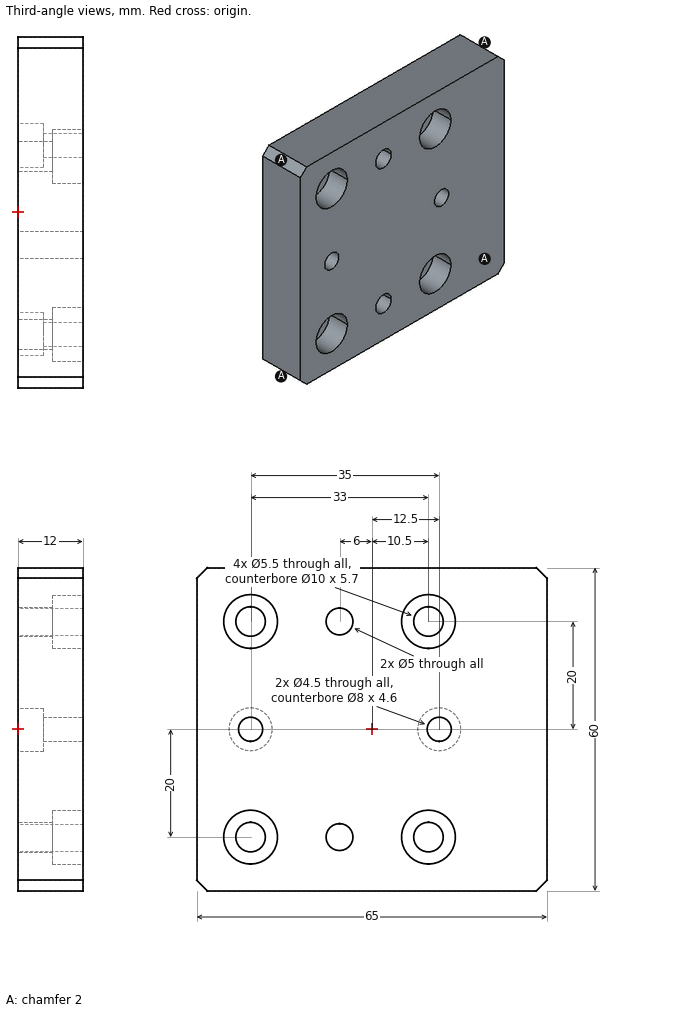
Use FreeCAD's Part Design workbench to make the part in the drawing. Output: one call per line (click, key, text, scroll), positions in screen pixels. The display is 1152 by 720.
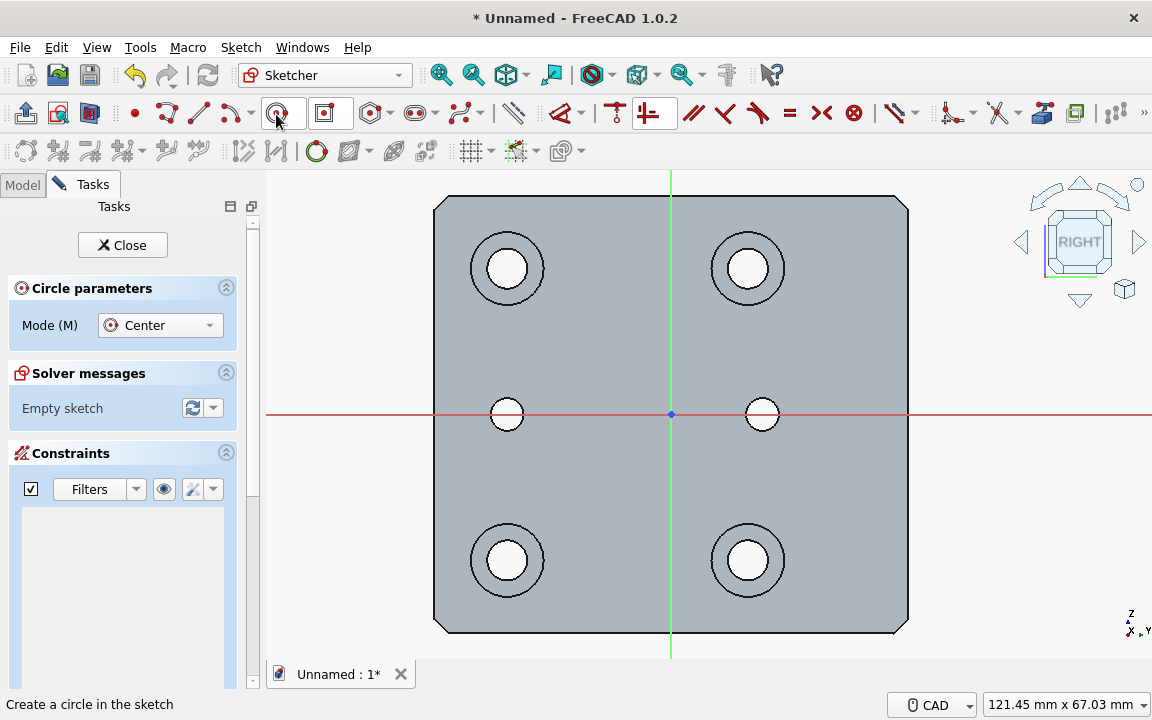
scroll(628, 269, up, 2)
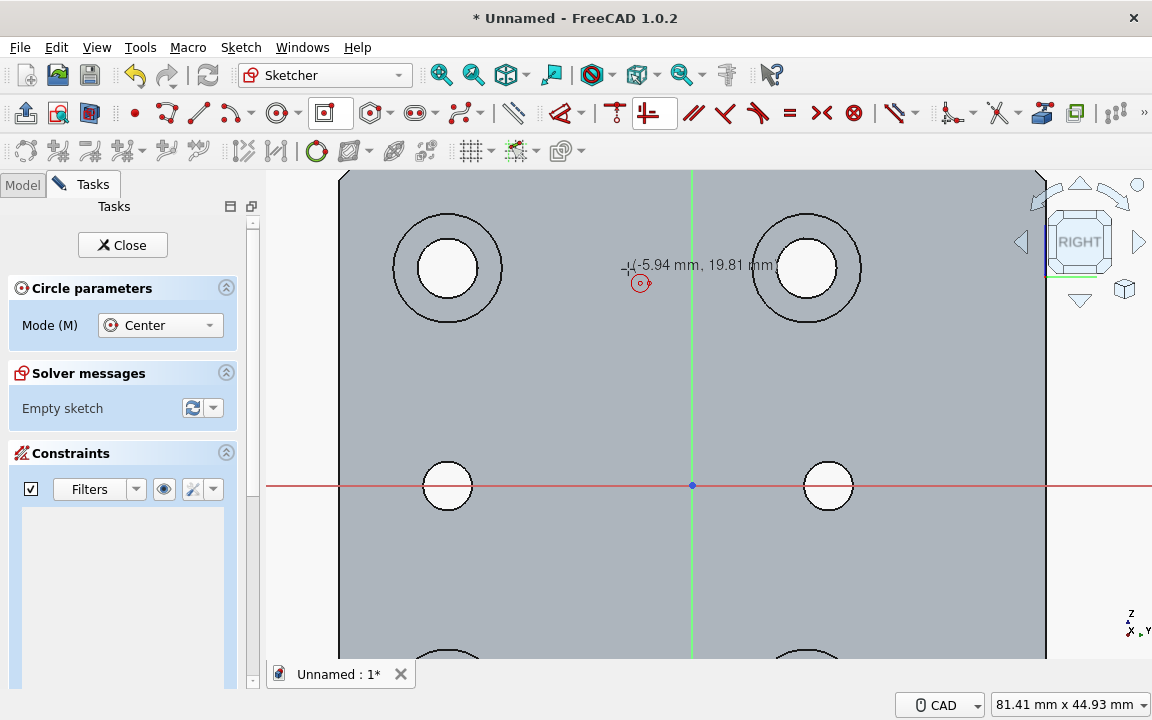
click(627, 268)
click(646, 249)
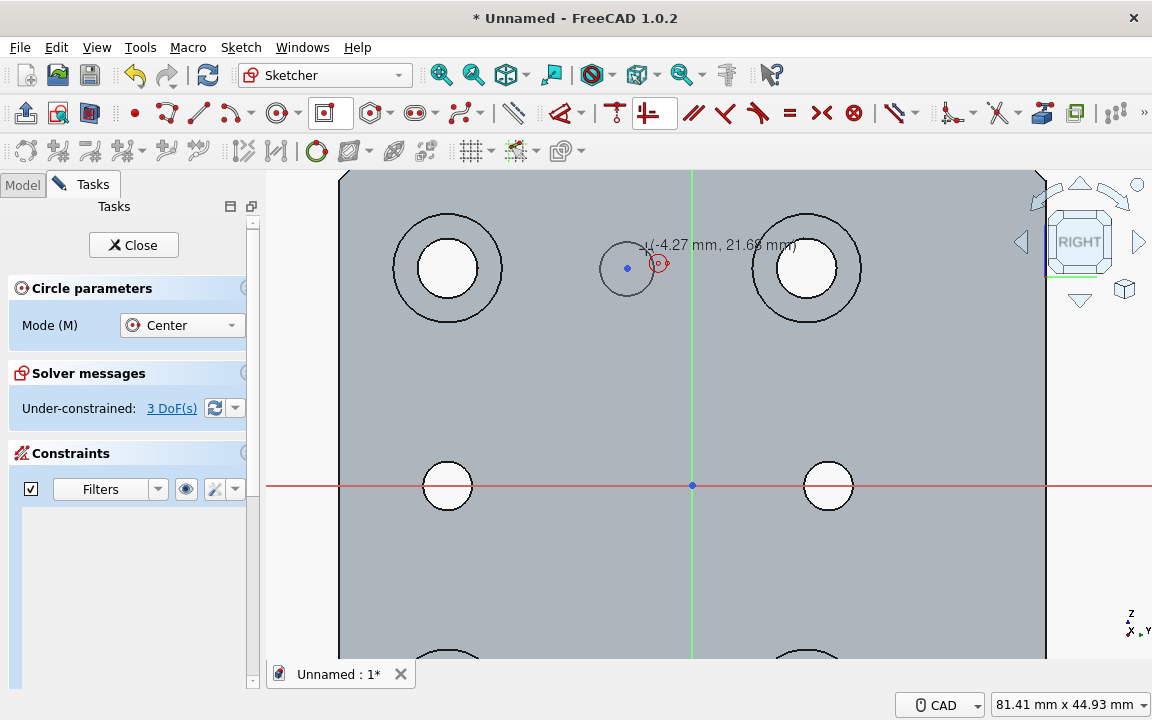
scroll(629, 269, down, 2)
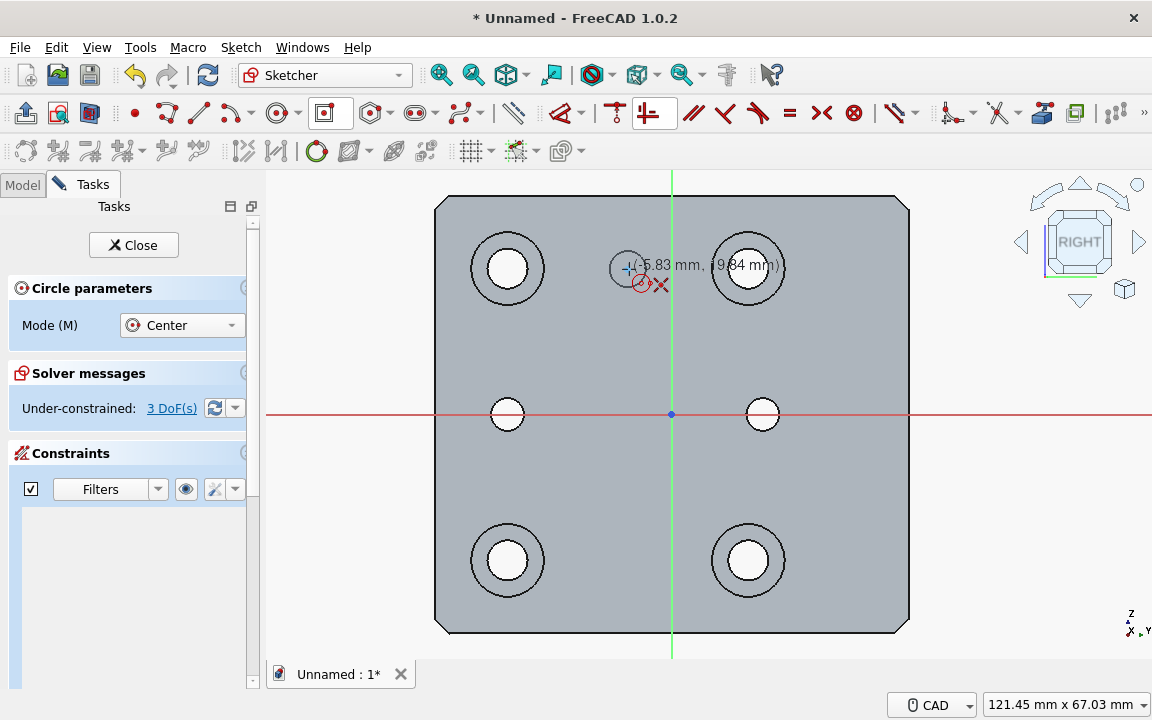
scroll(628, 560, up, 2)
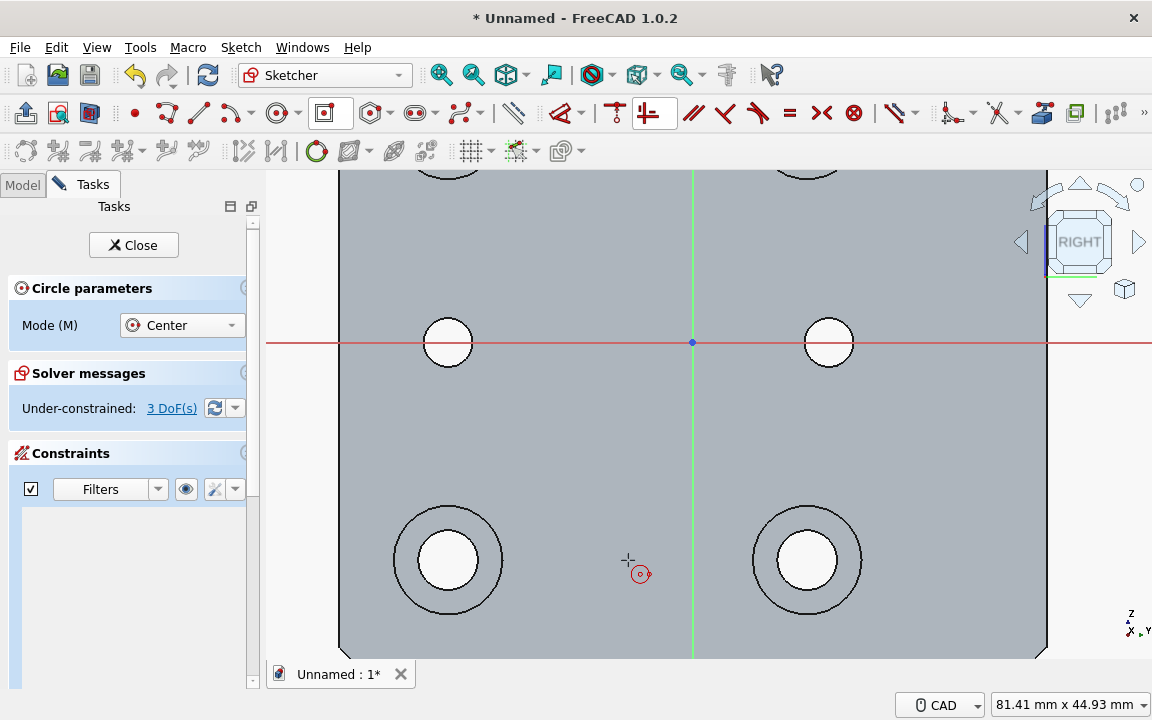
click(628, 560)
click(647, 541)
key(Escape)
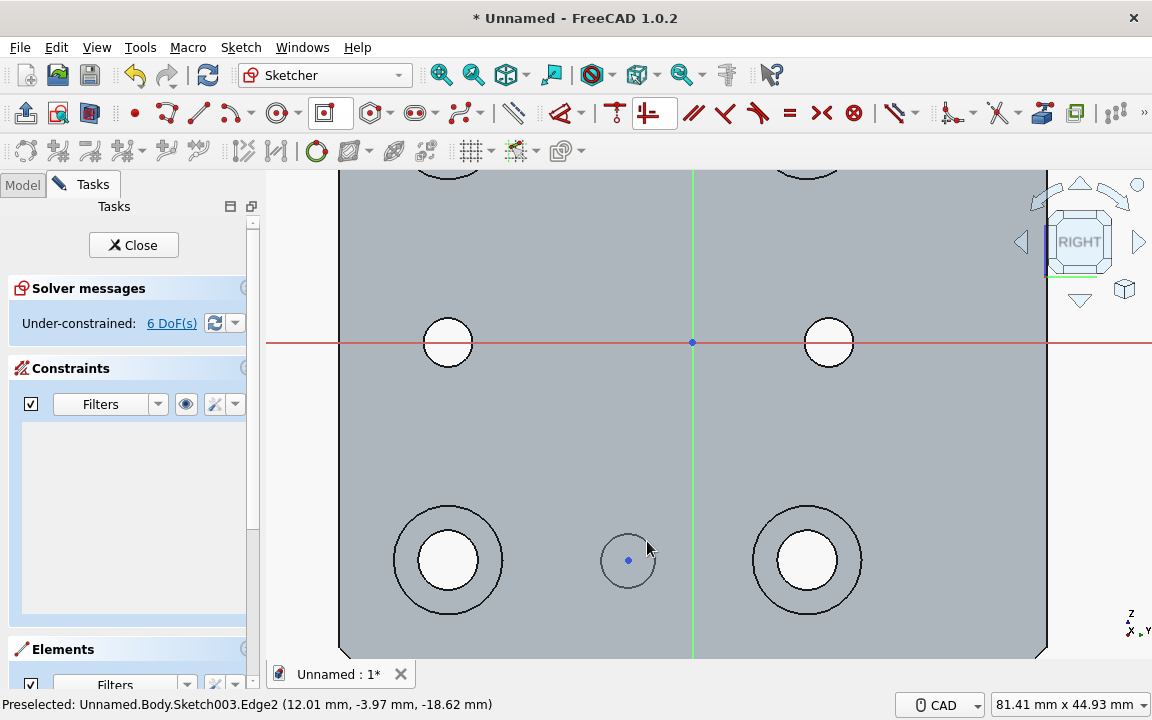
scroll(628, 561, down, 2)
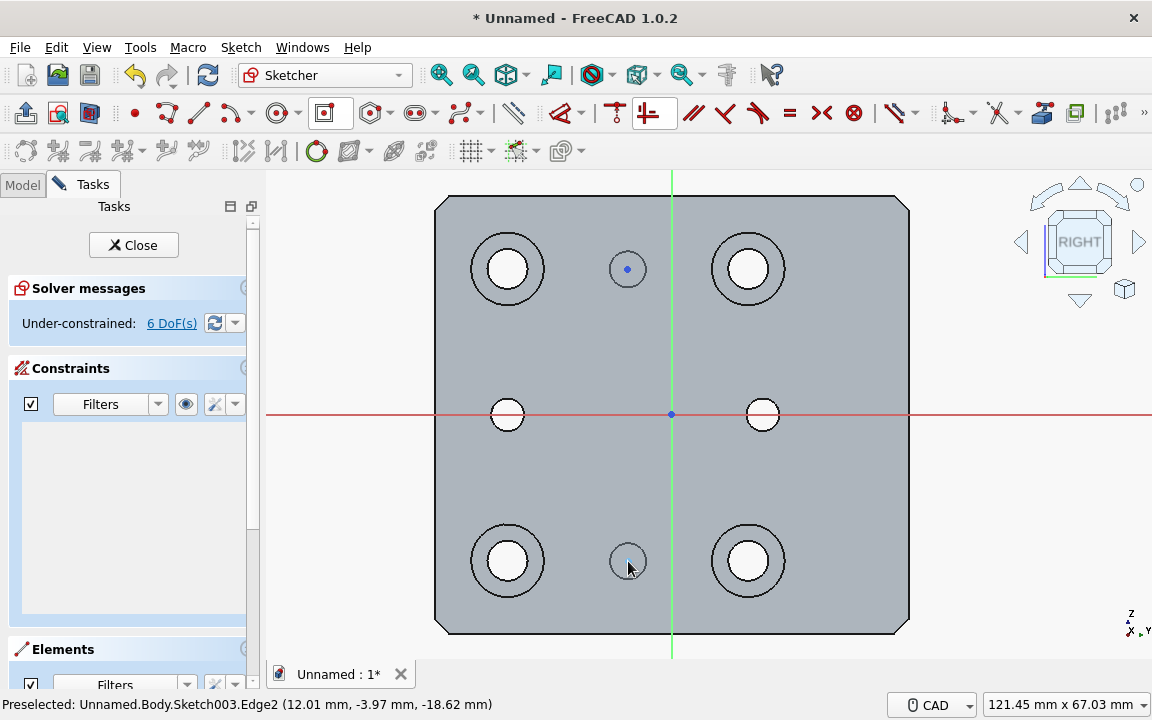
click(640, 257)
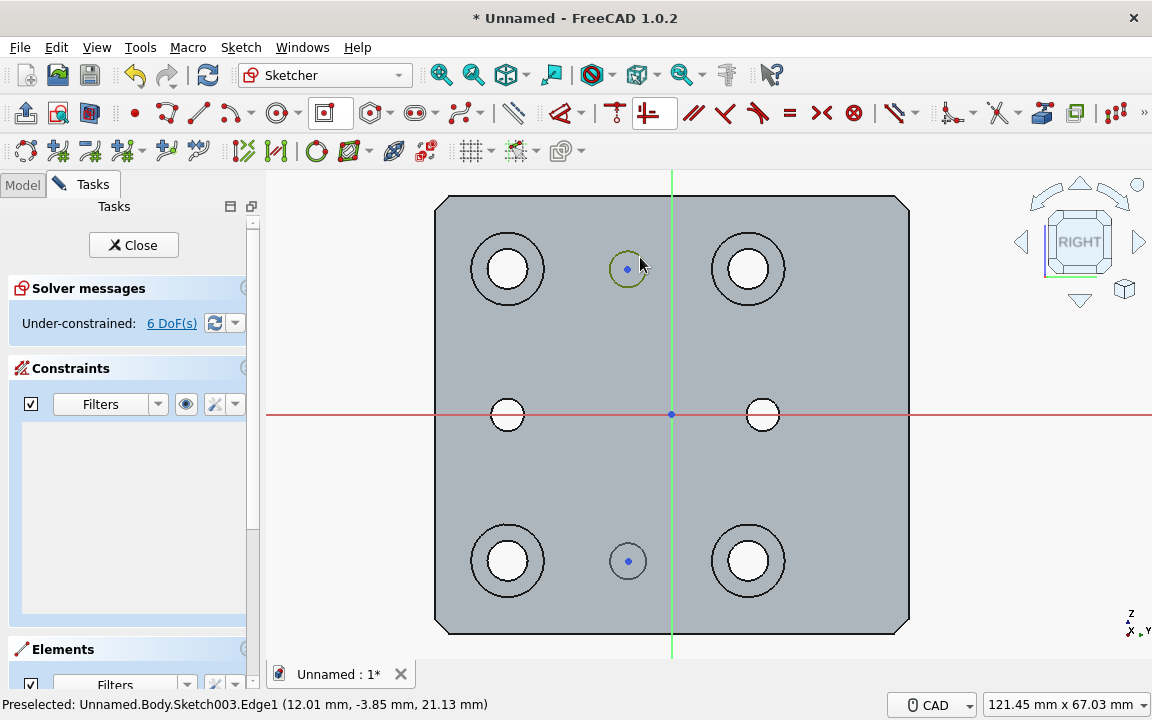
click(641, 548)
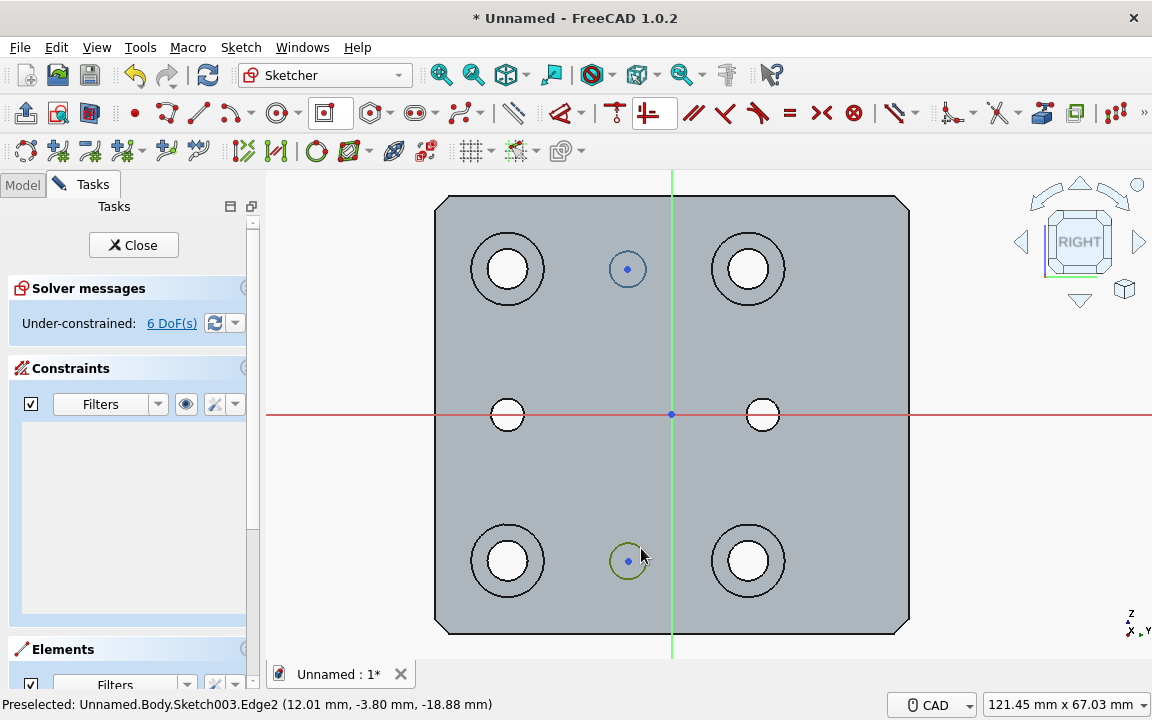
click(790, 114)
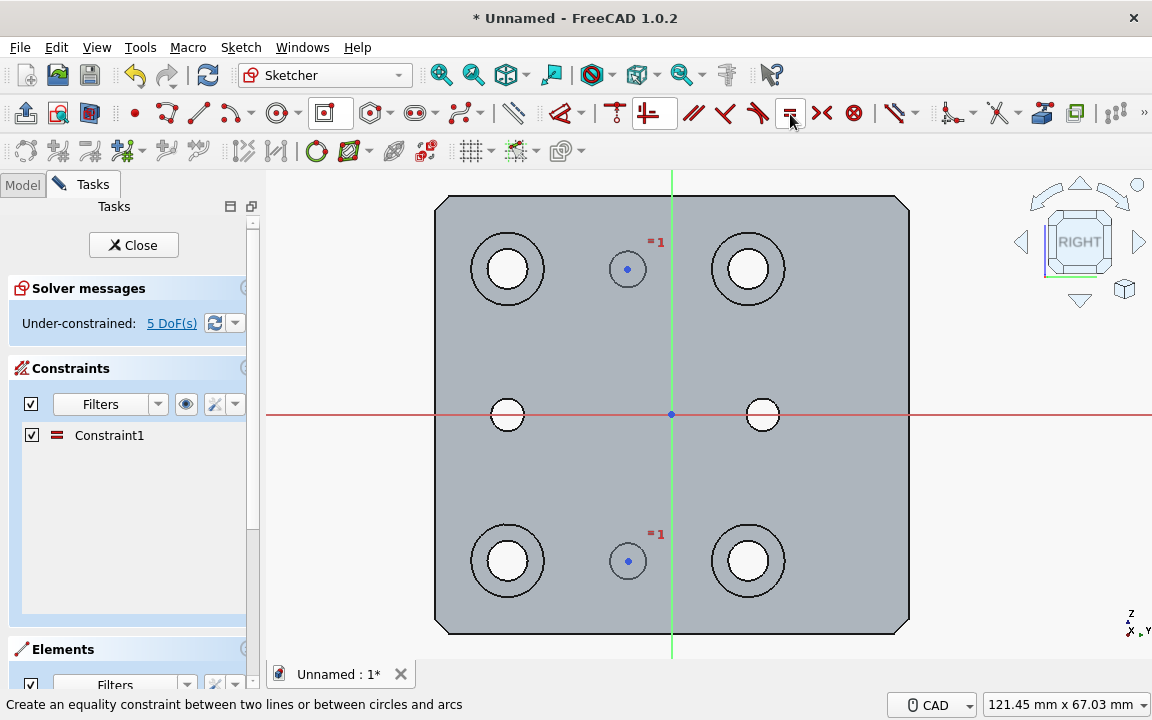
click(628, 269)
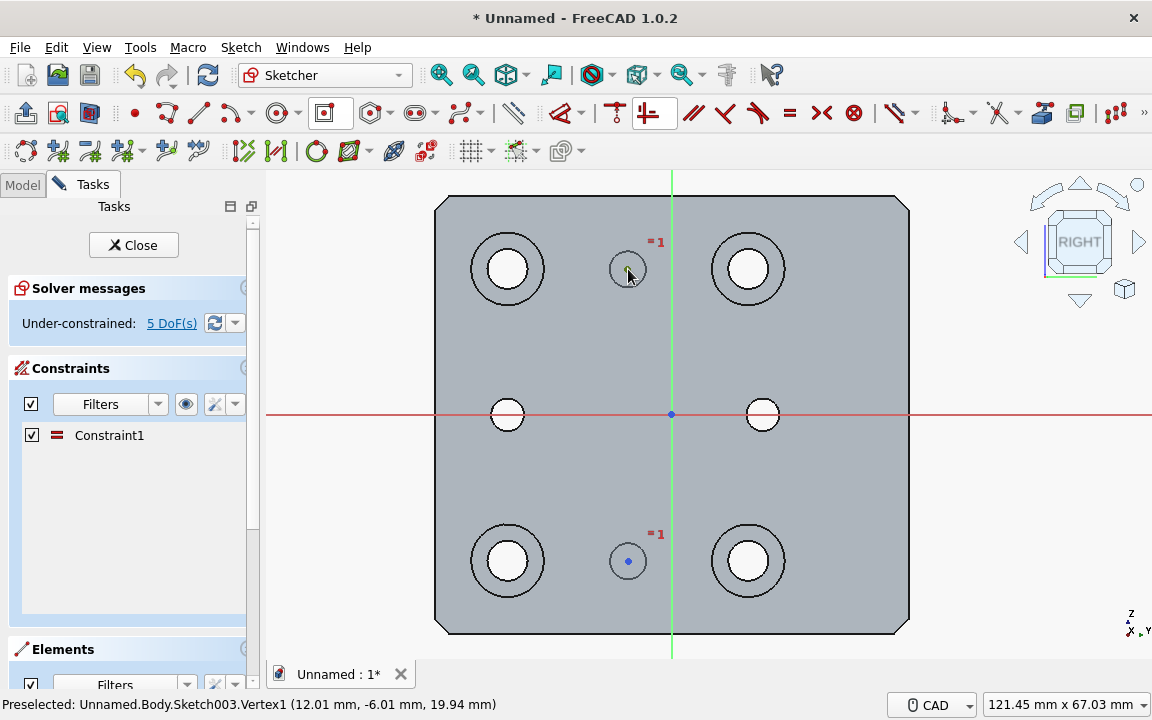
click(628, 561)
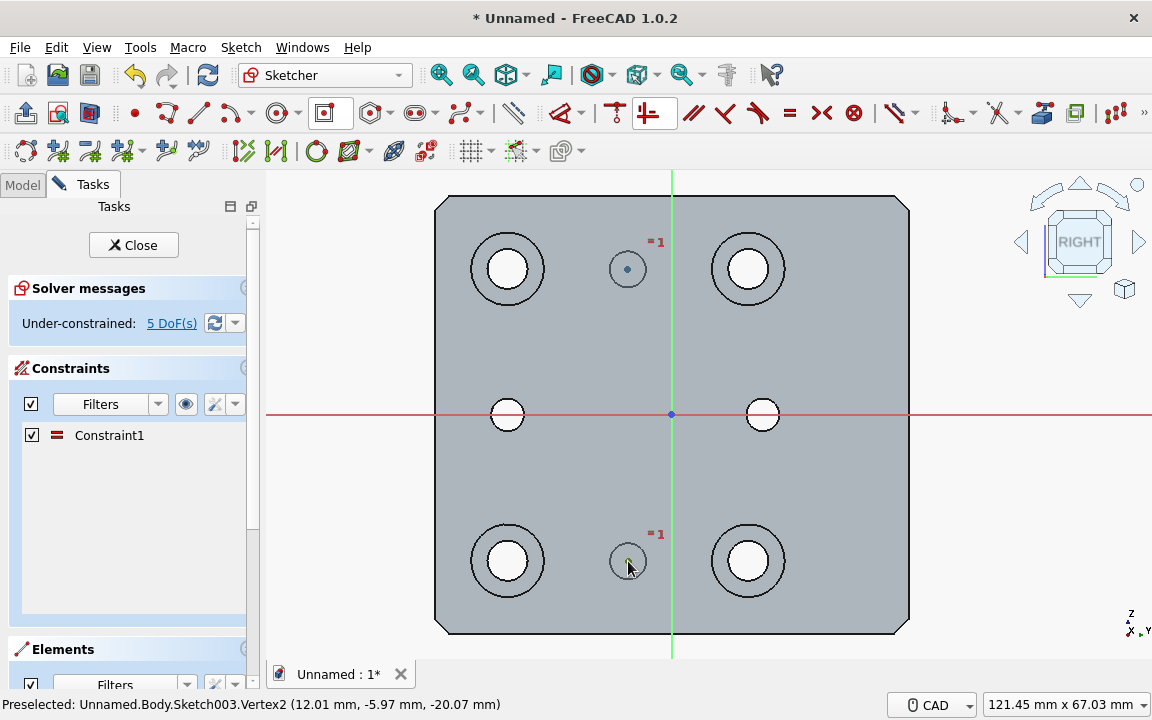
click(672, 114)